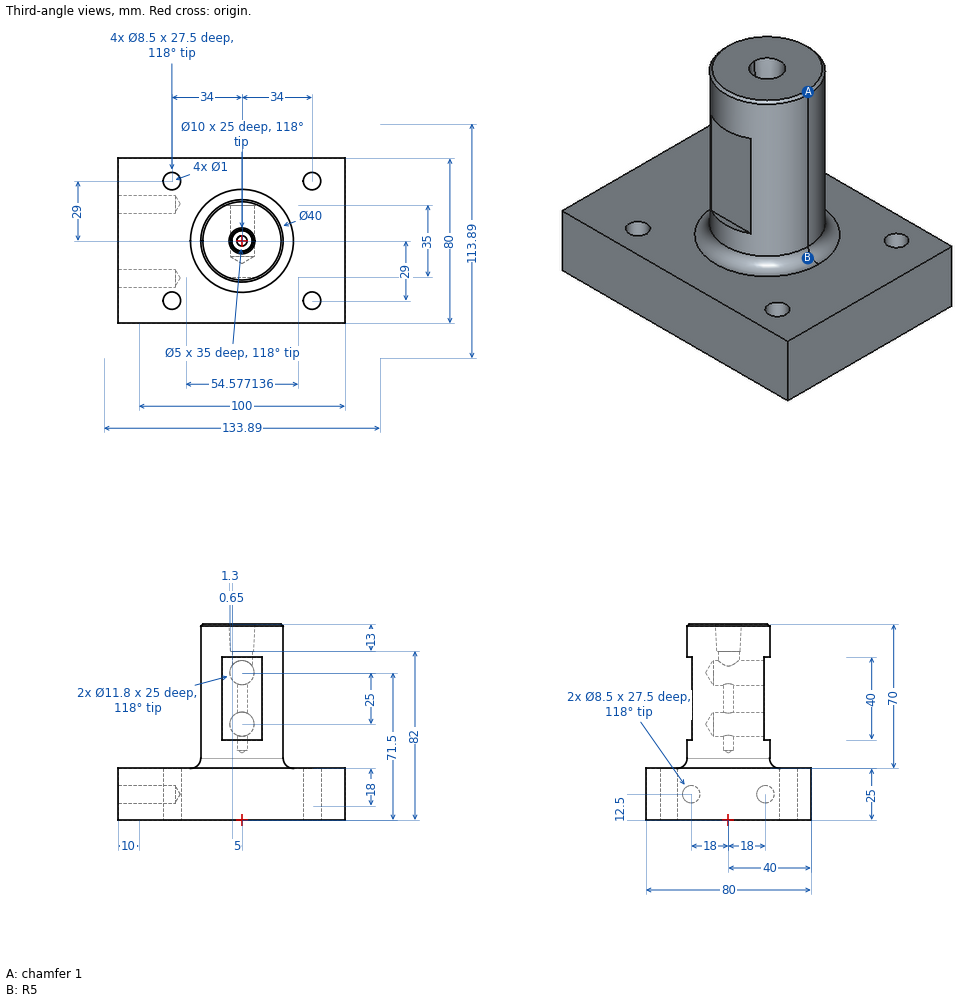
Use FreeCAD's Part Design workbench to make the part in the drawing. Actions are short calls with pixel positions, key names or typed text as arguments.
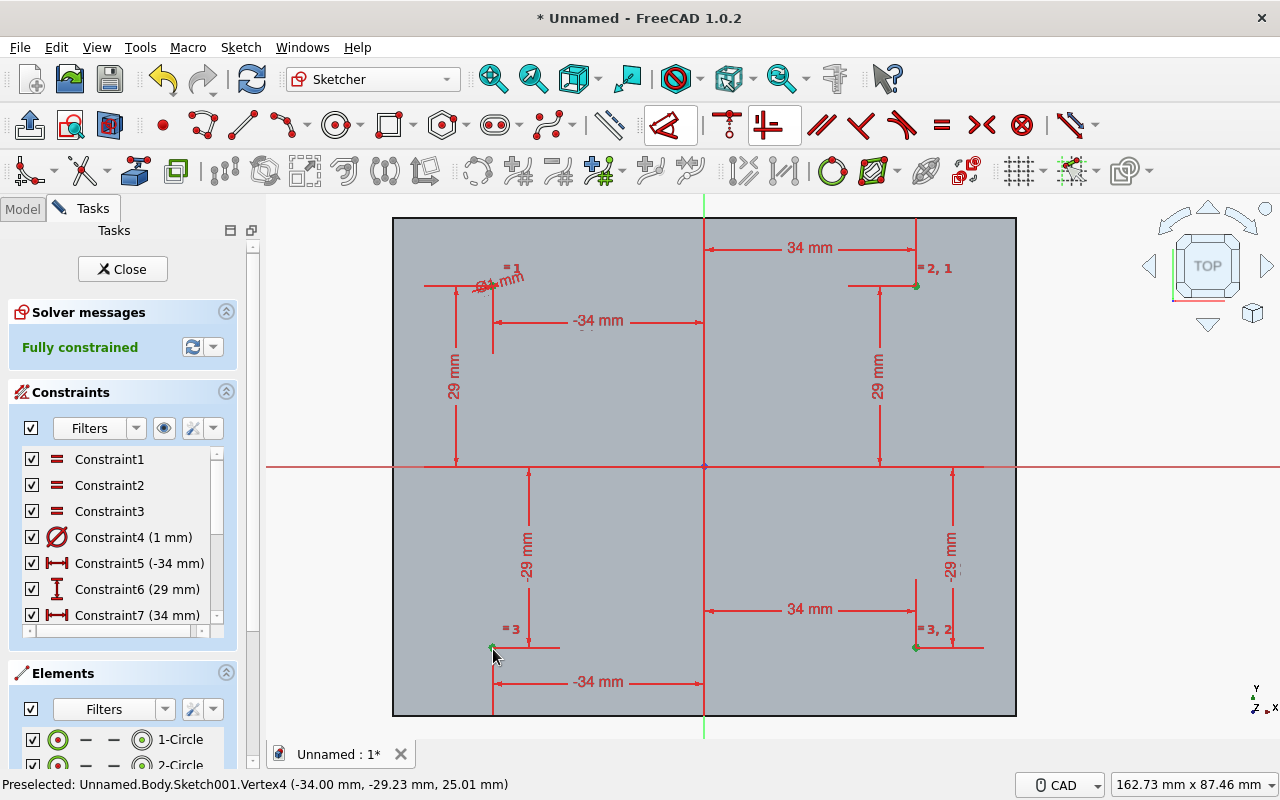
click(123, 269)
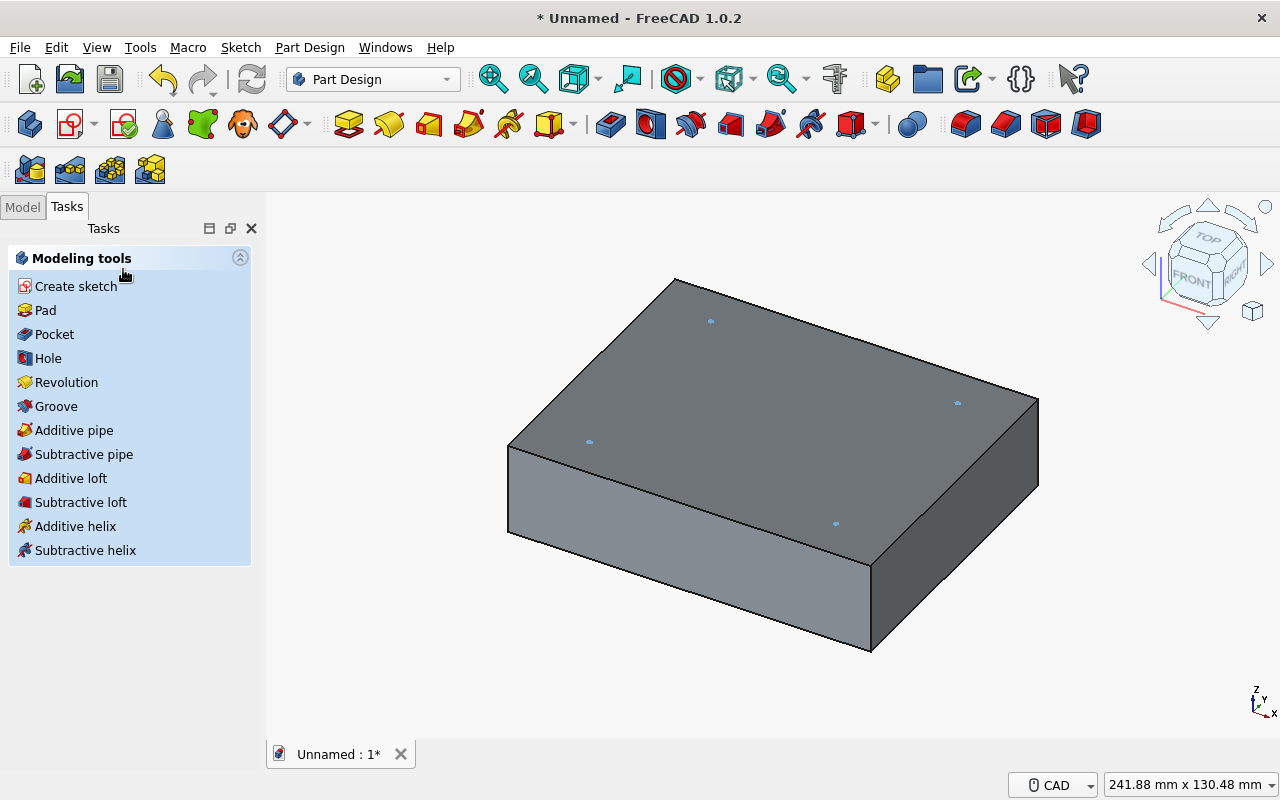
click(612, 124)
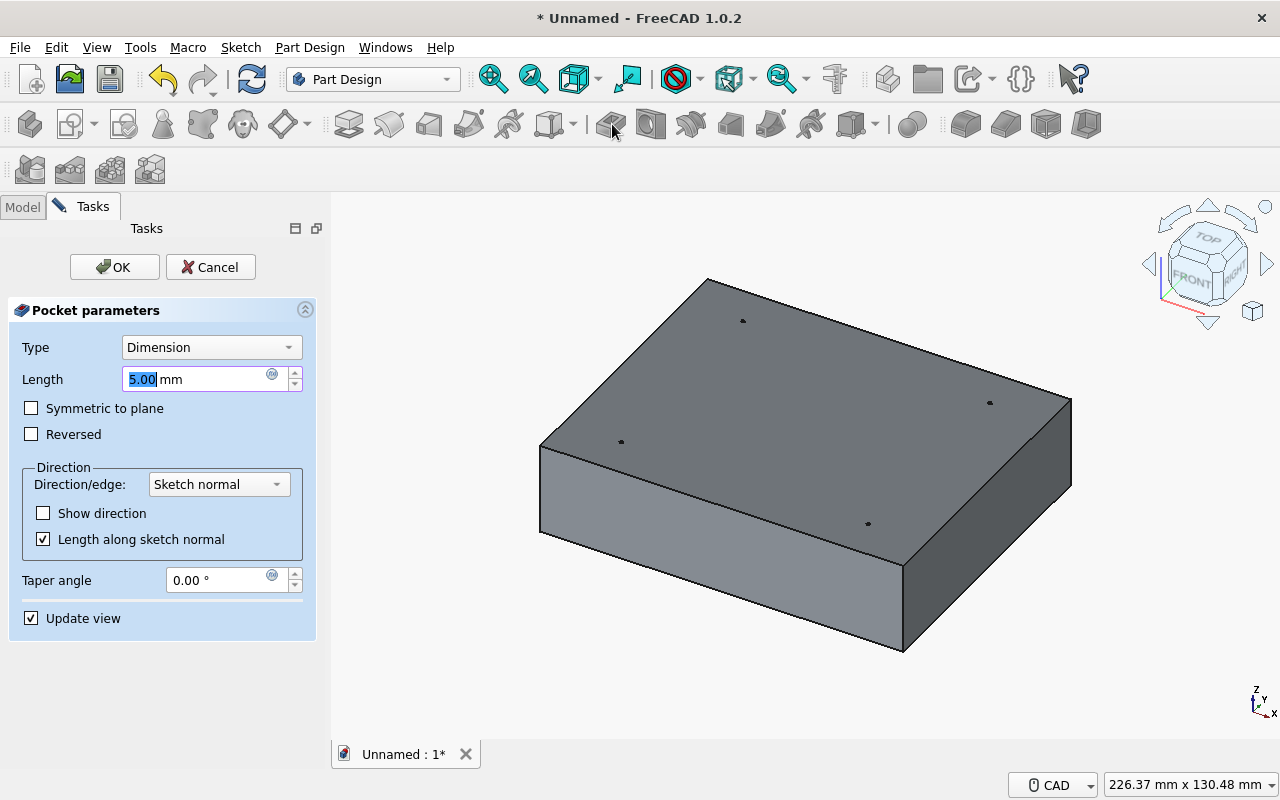
text(18)
key(Tab)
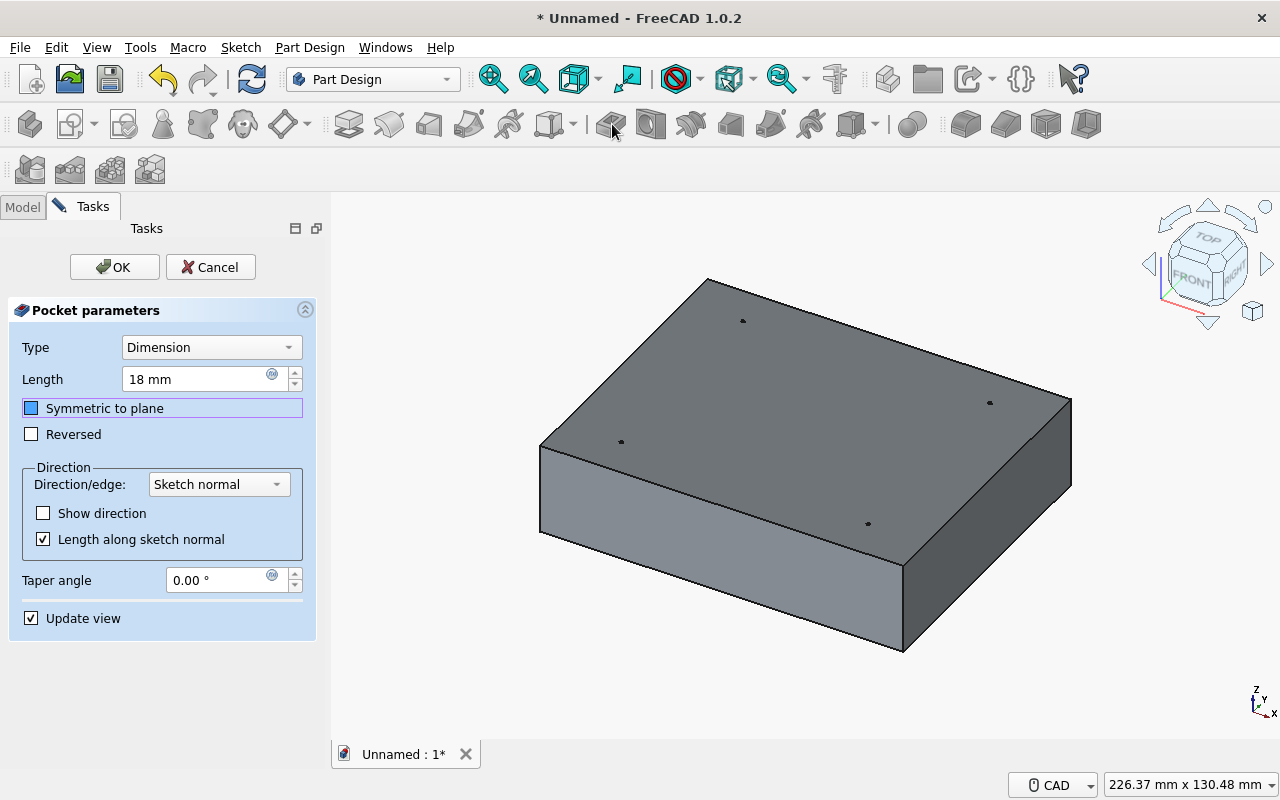
click(115, 267)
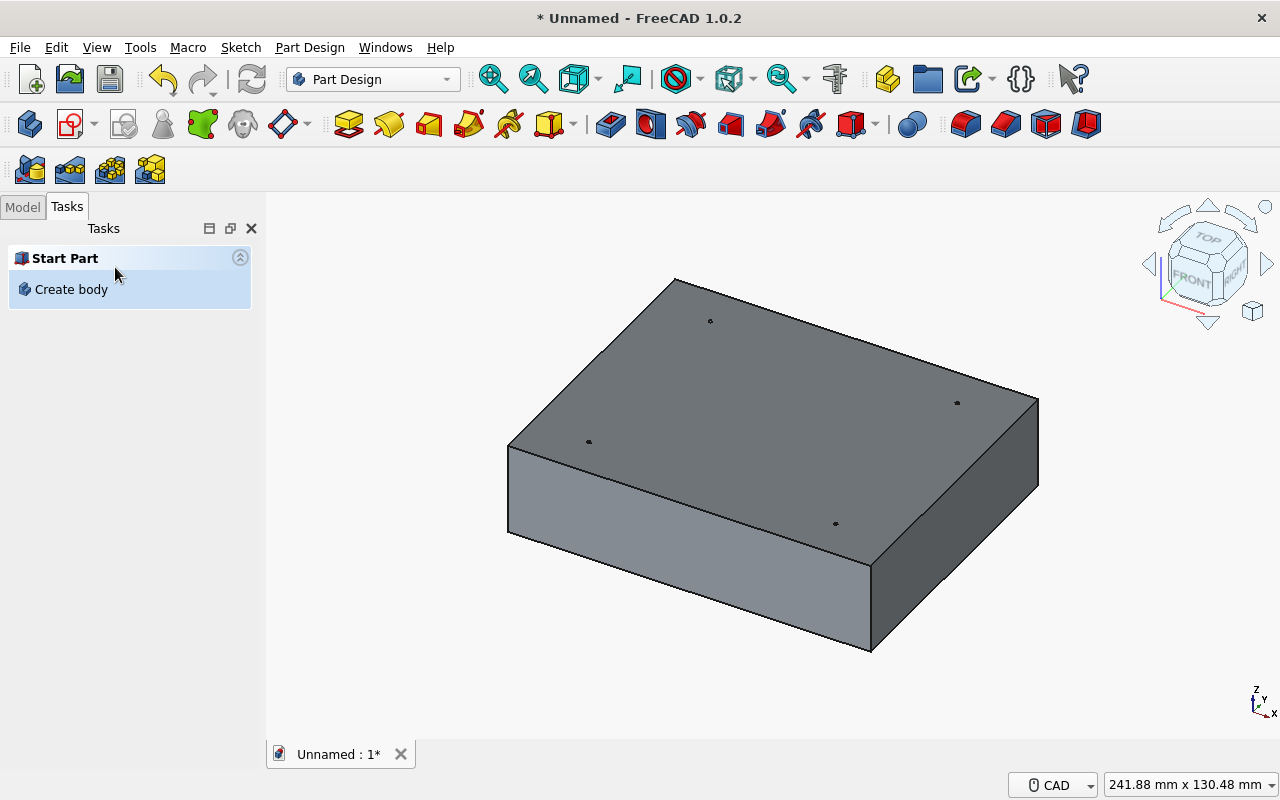
click(773, 422)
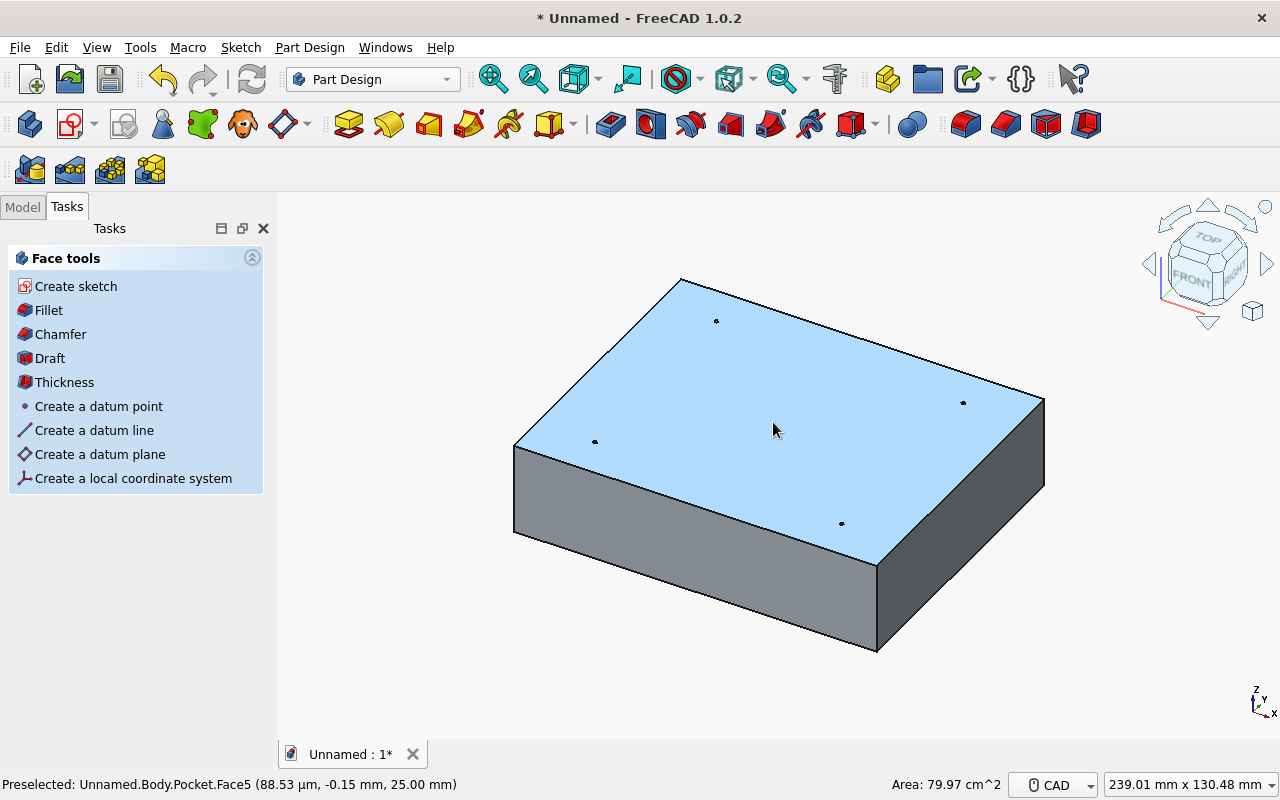
click(70, 124)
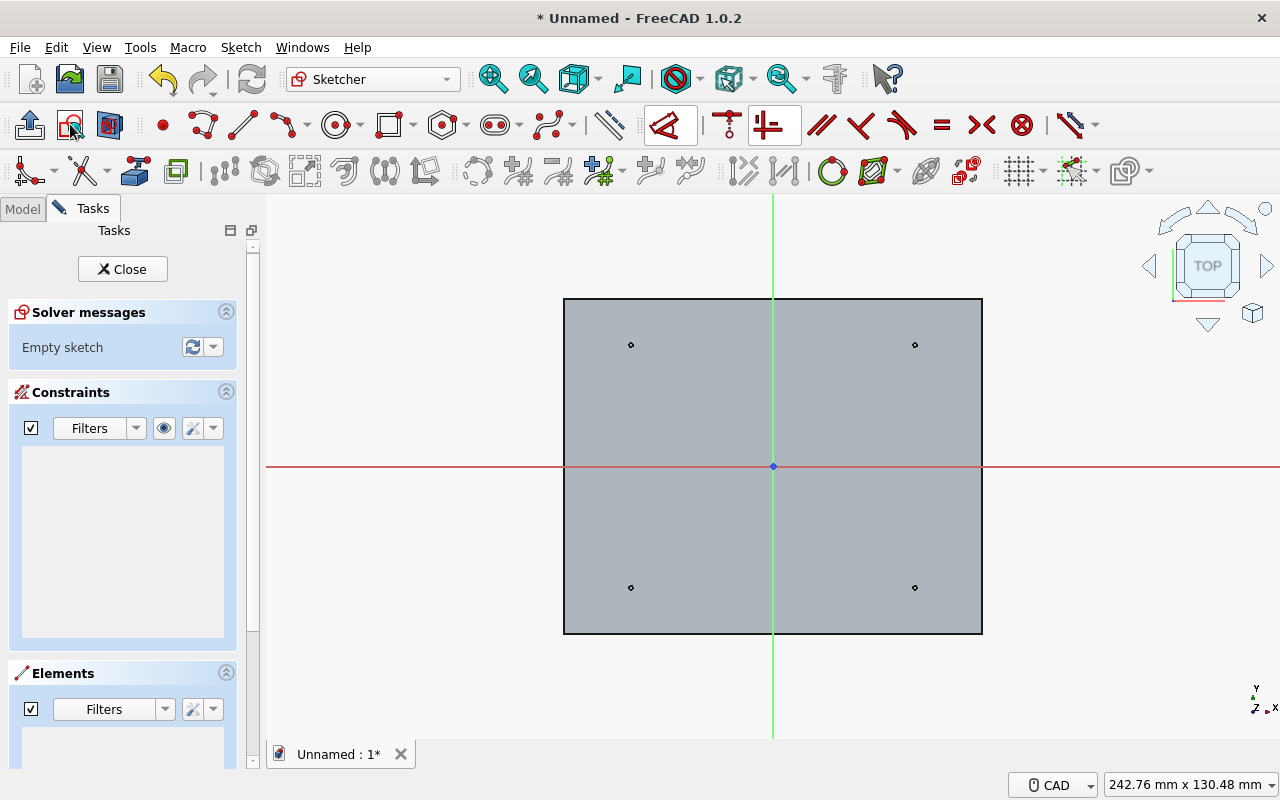
scroll(829, 467, up, 4)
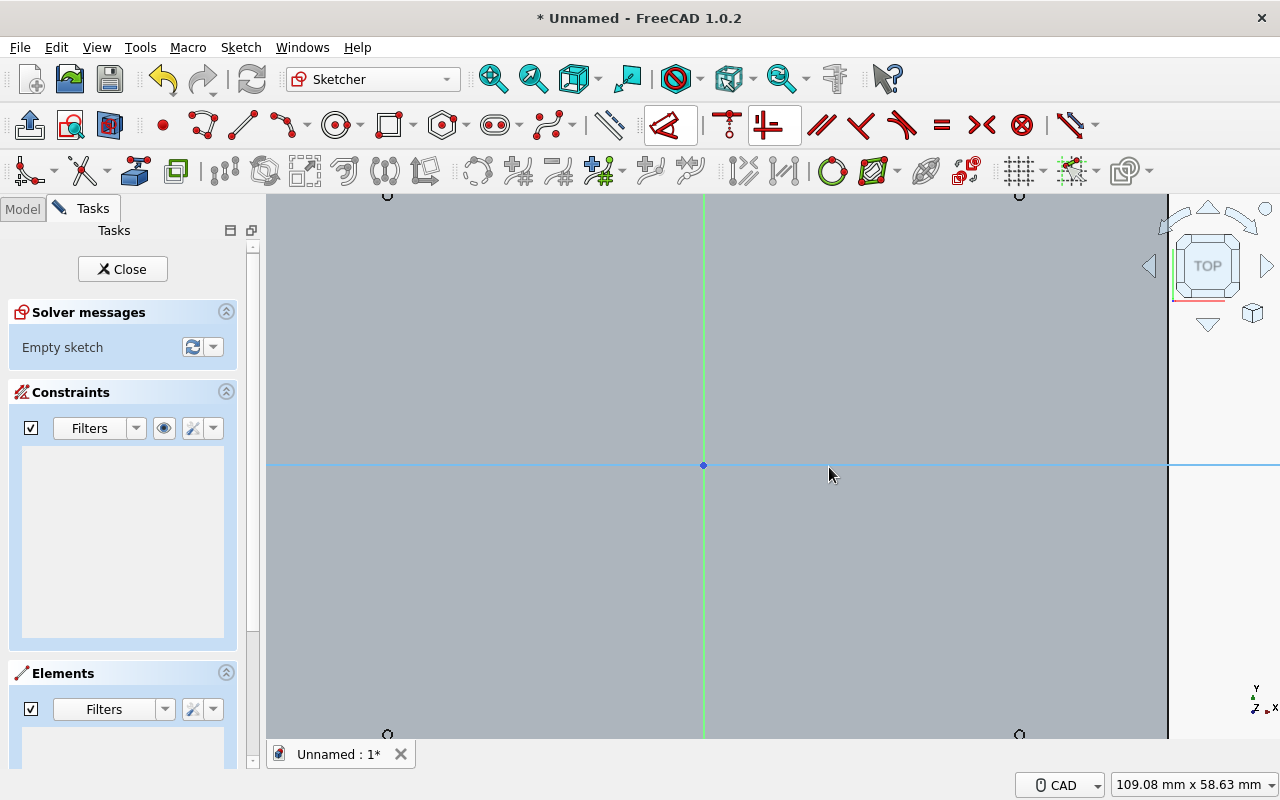
click(336, 126)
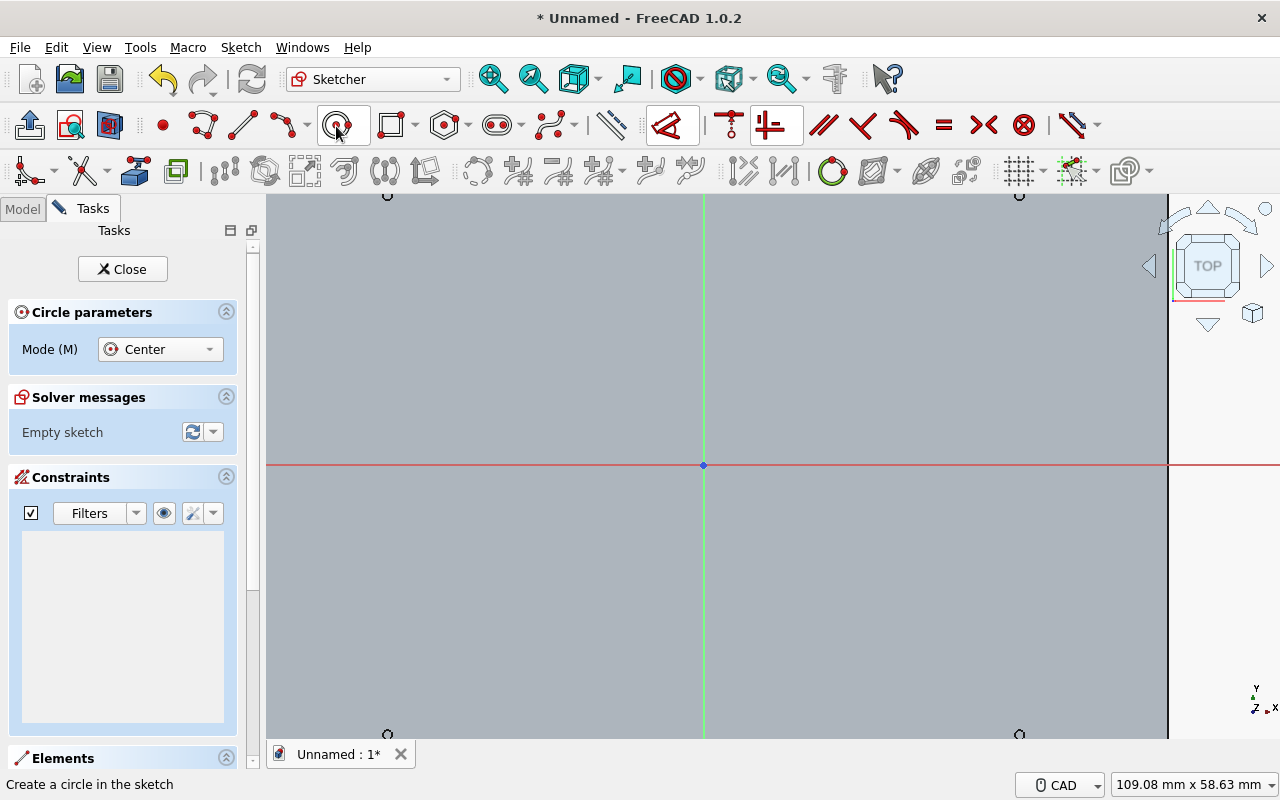
click(704, 465)
click(835, 334)
key(Escape)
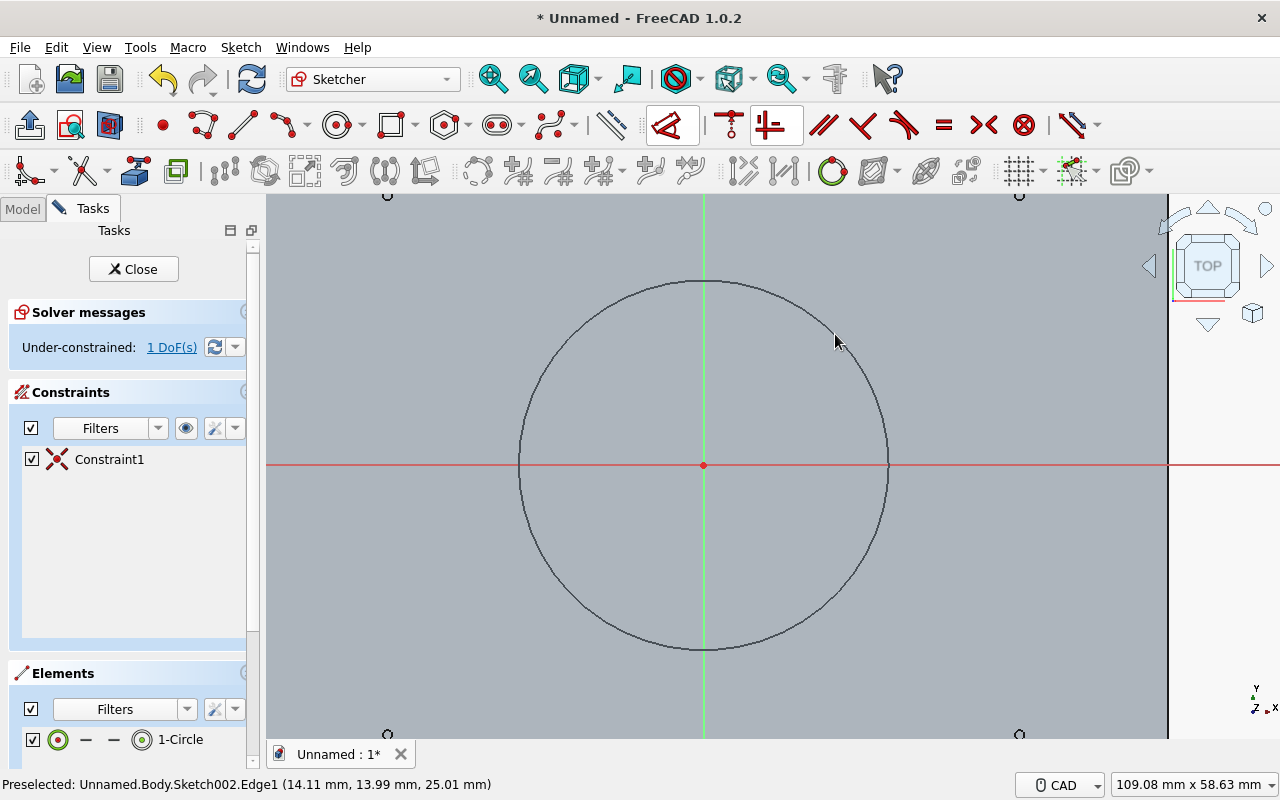
click(834, 334)